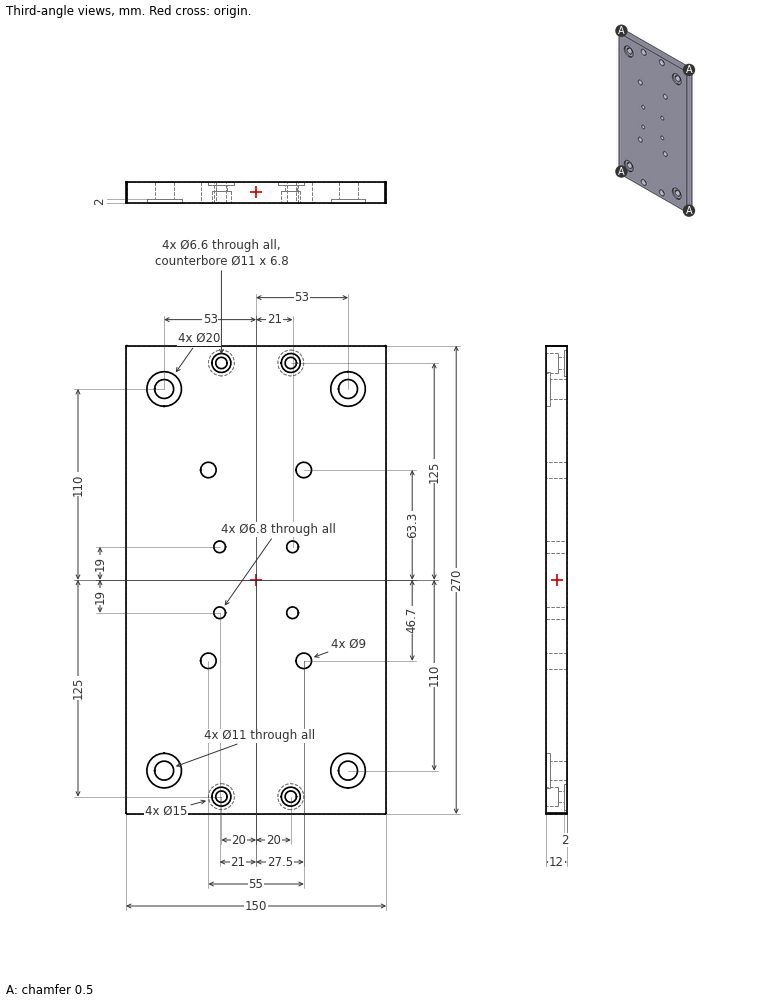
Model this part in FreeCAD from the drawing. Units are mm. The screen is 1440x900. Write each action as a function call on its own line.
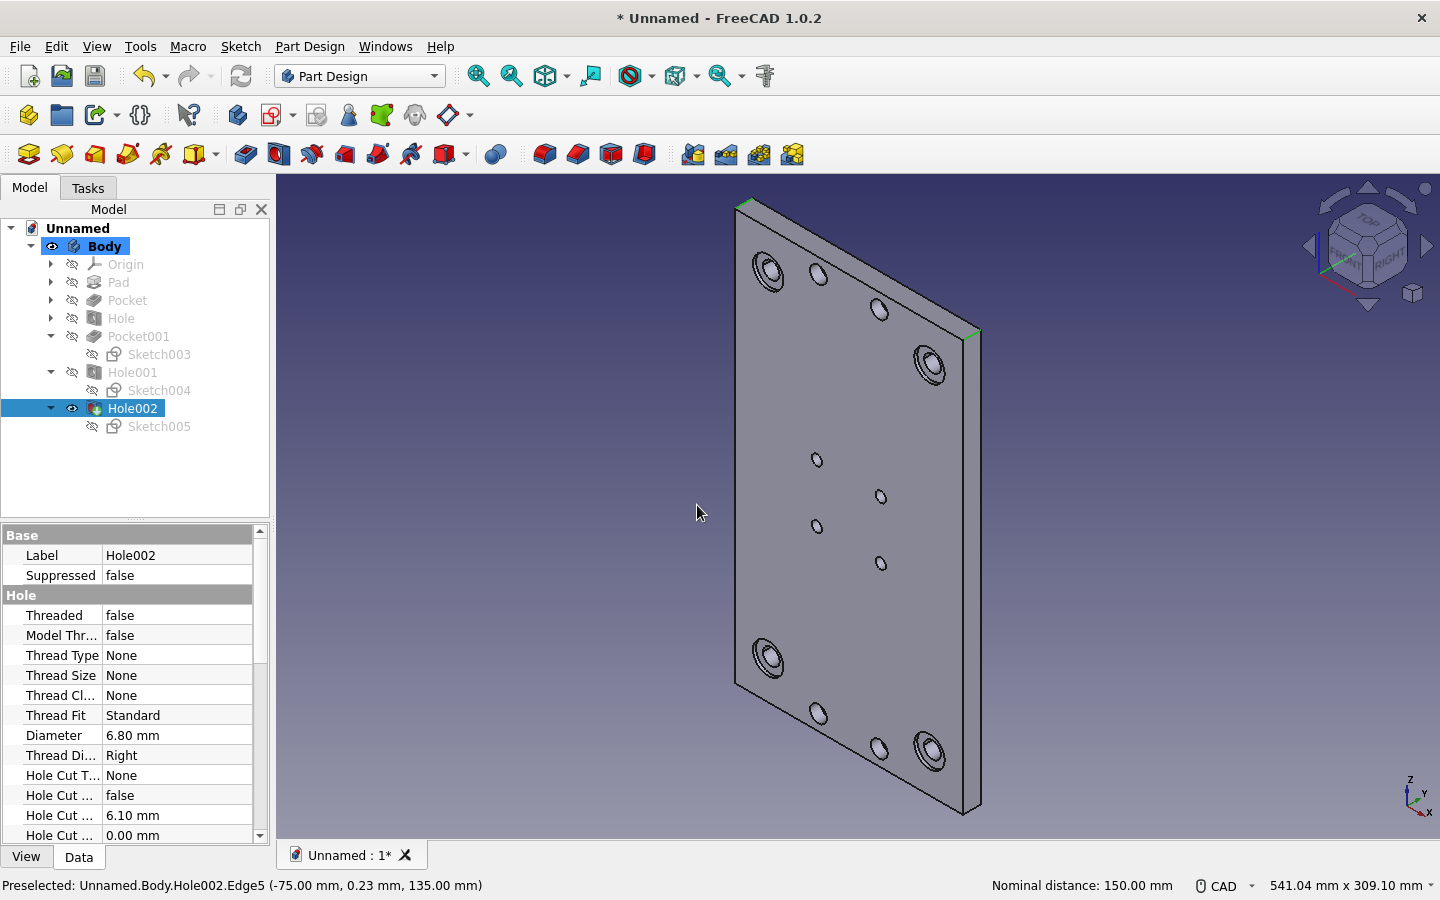
key(1)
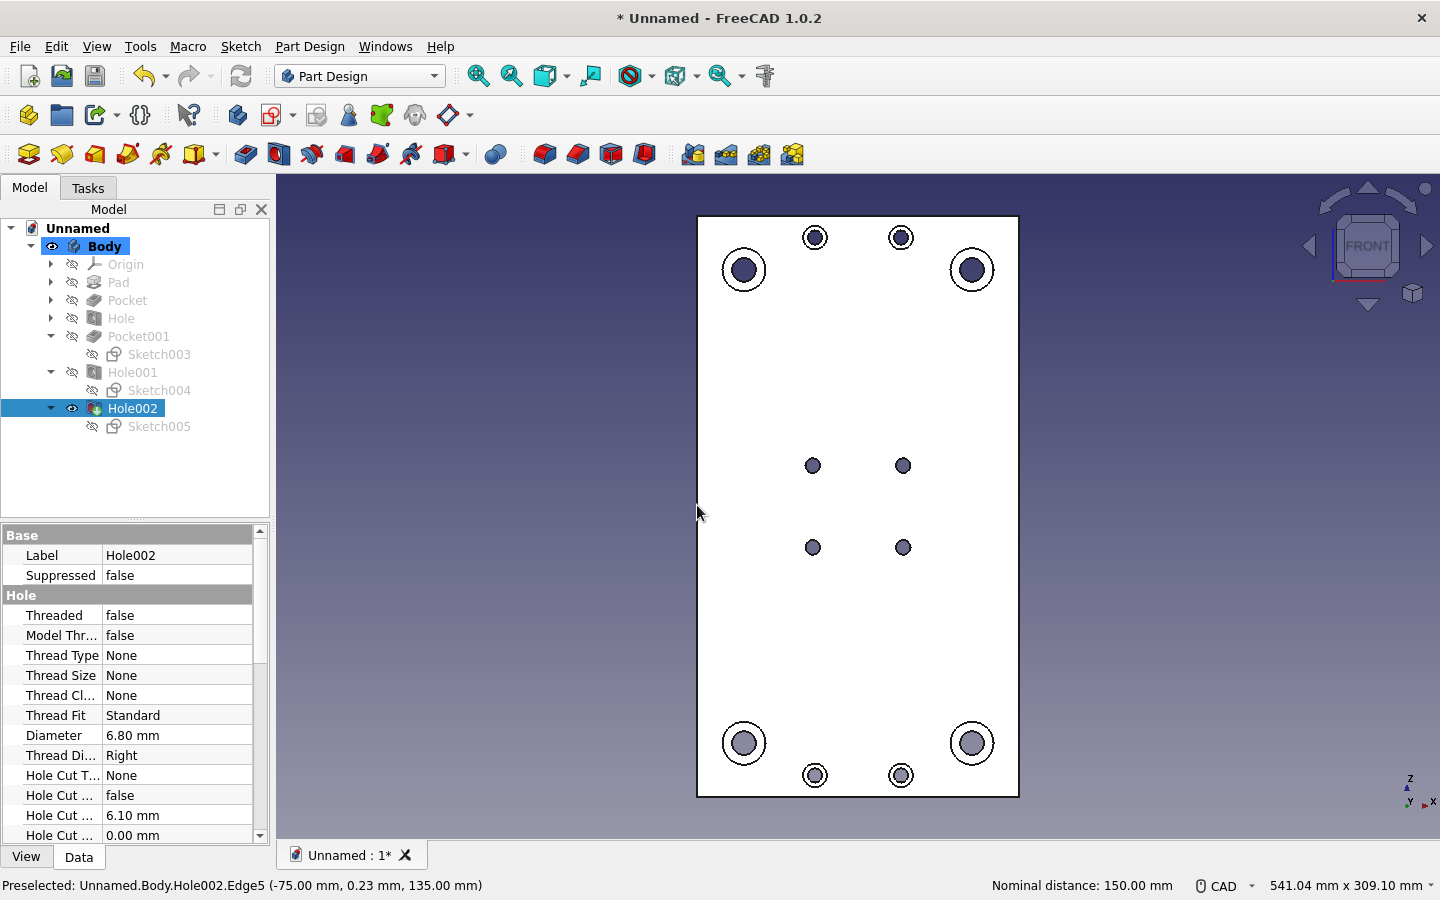
key(3)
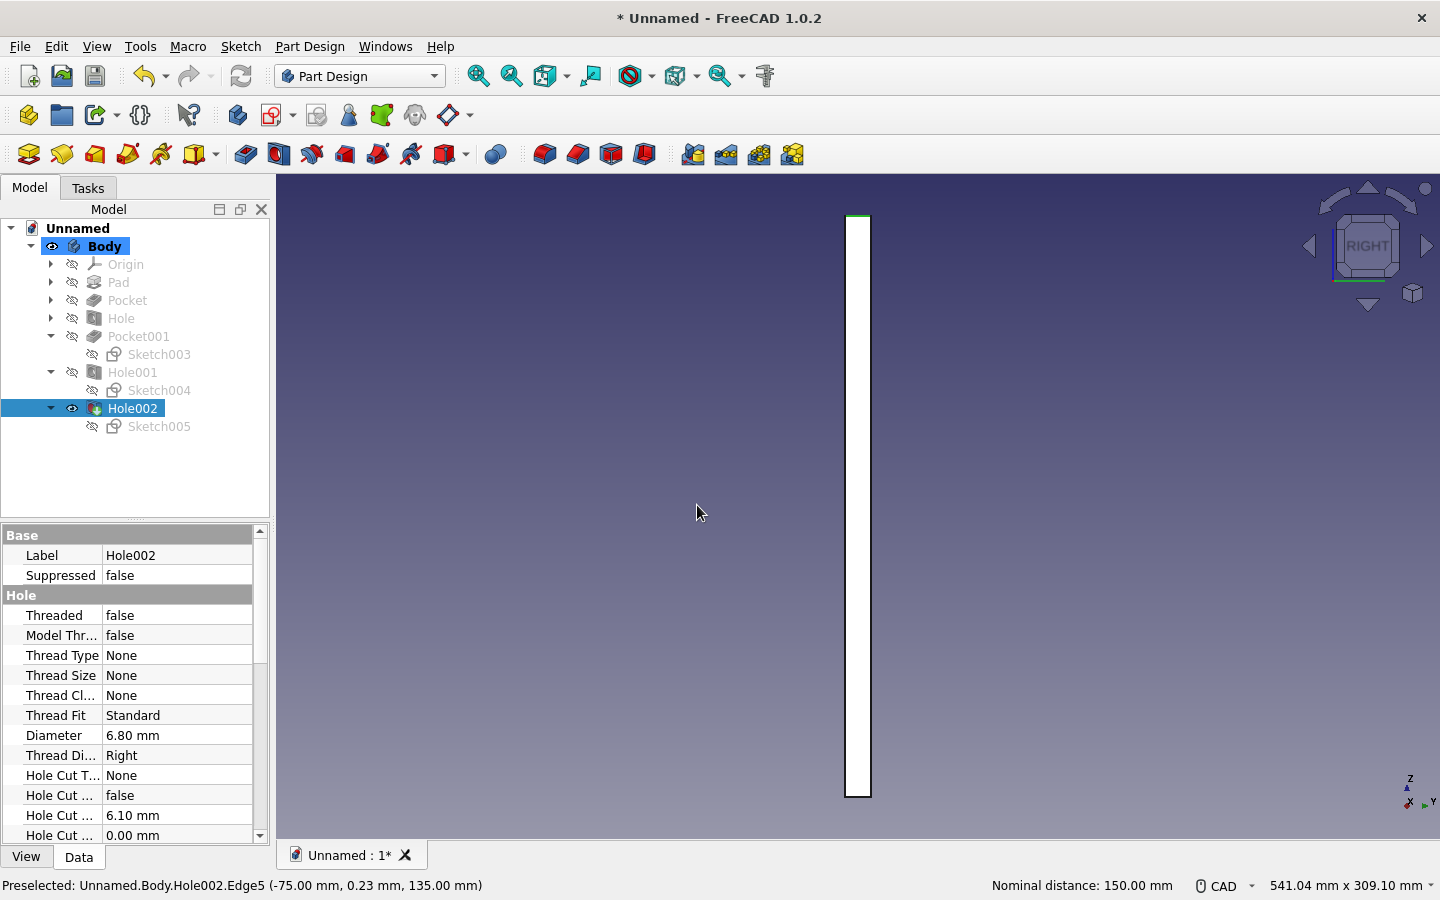
click(858, 796, ctrl)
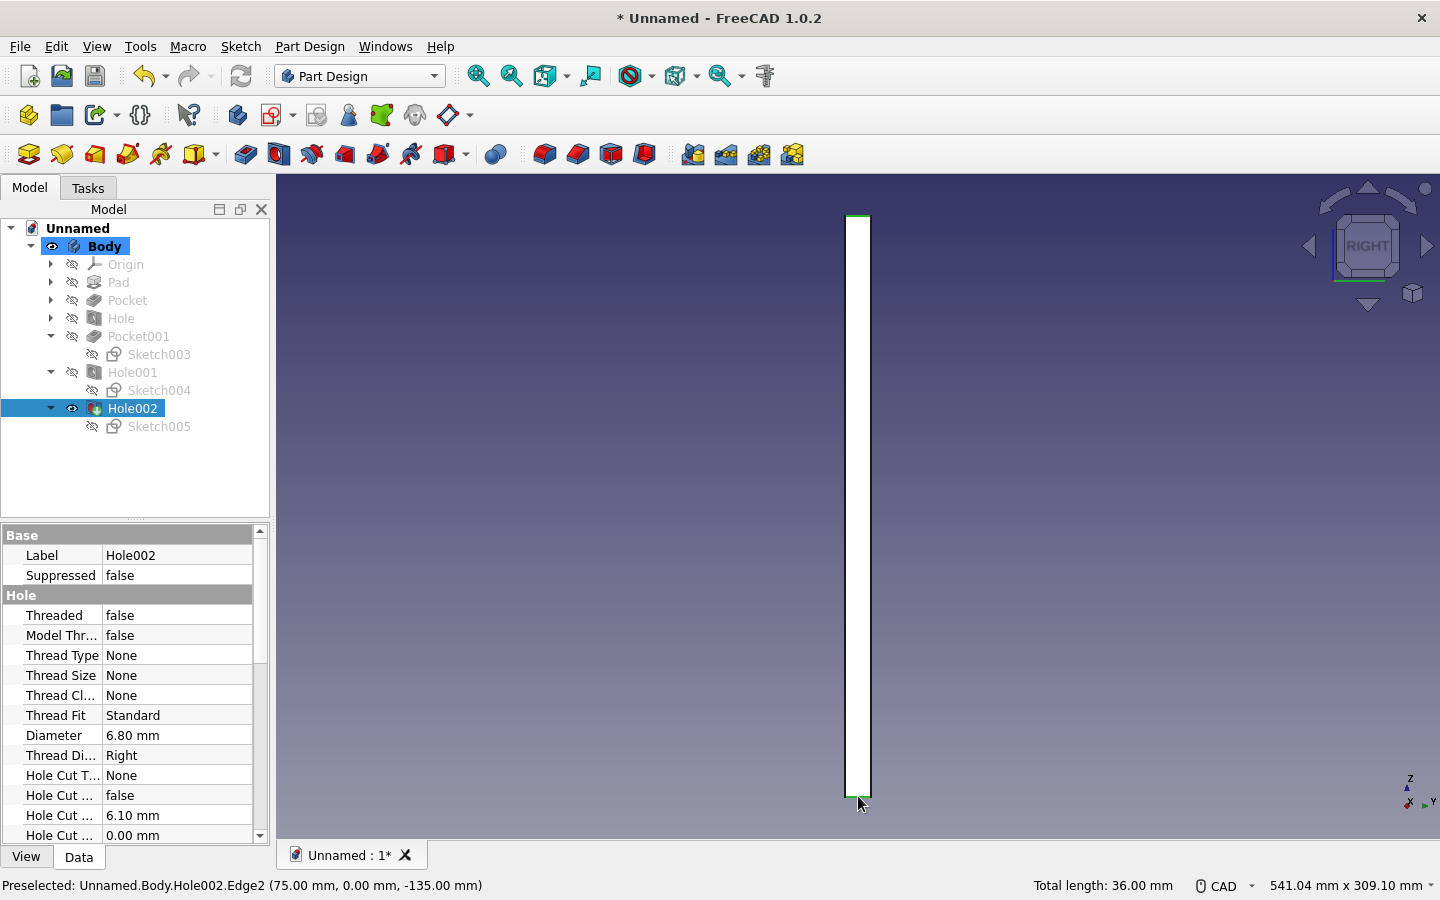
key(5)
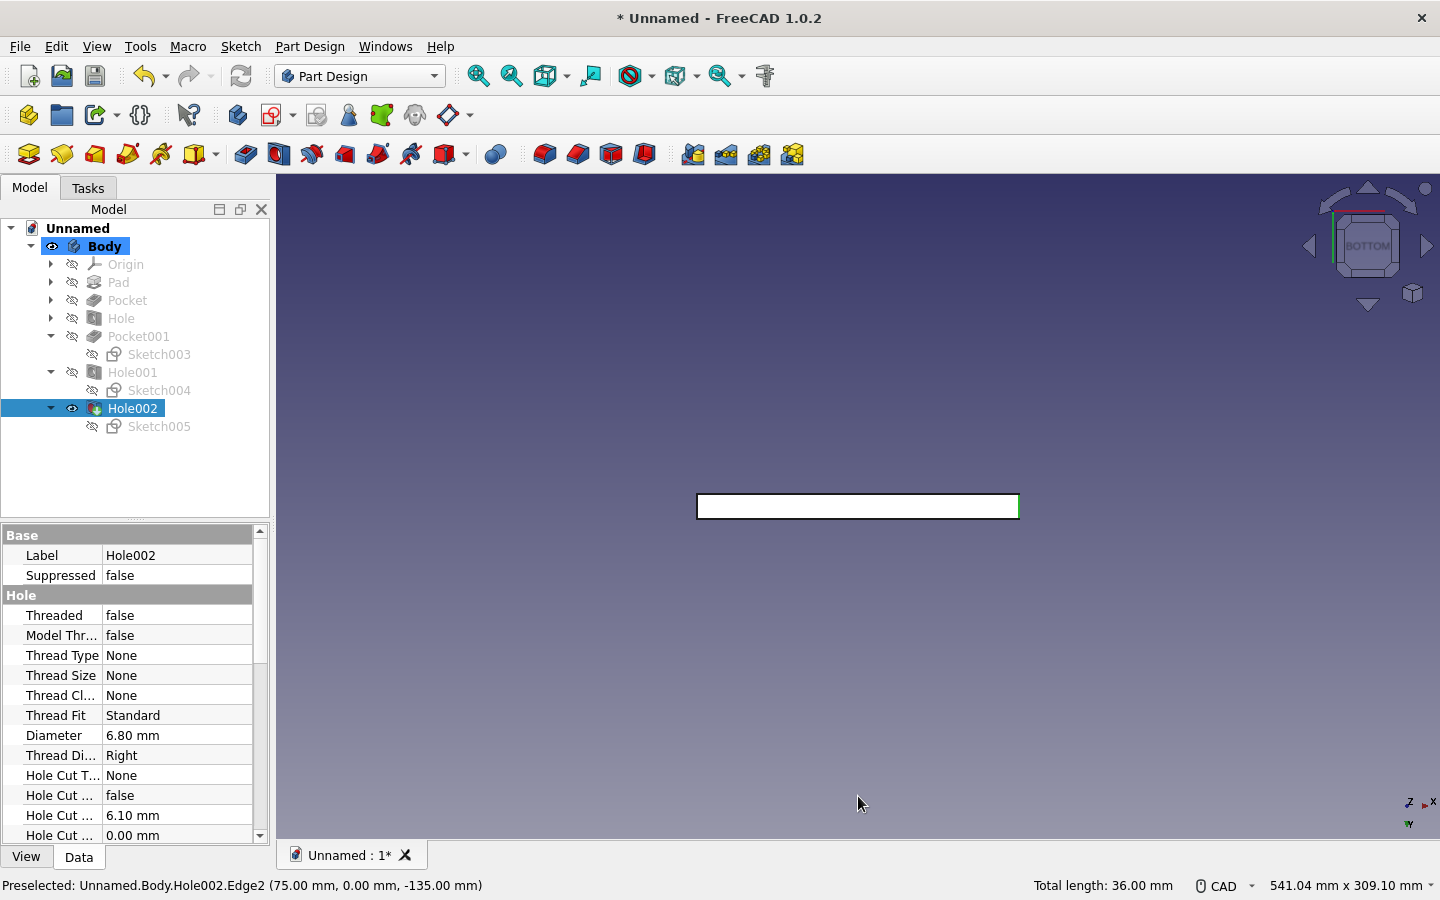
key(v)
key(f)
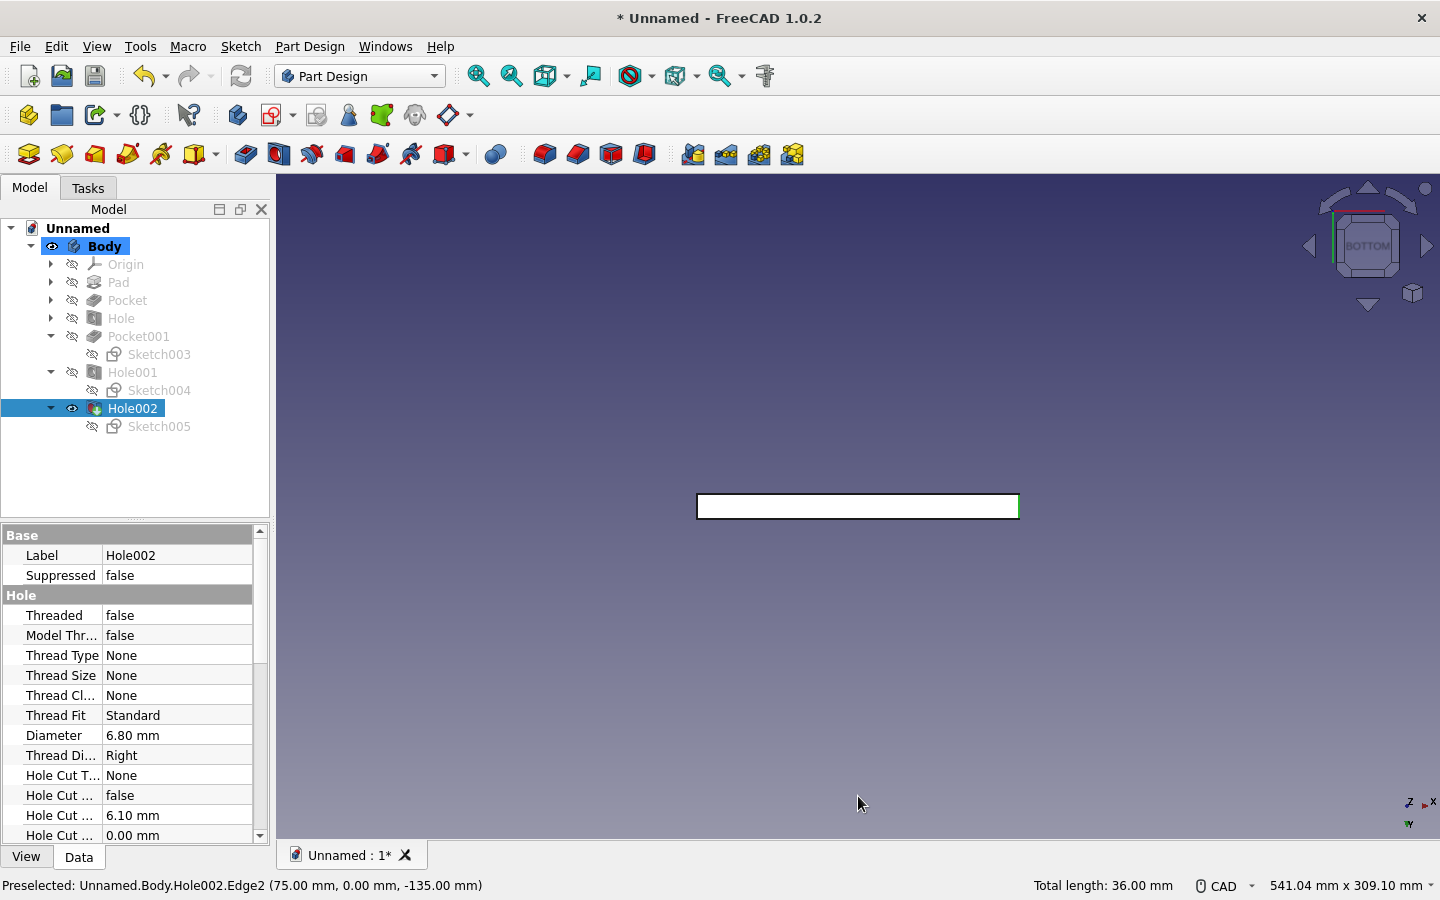
click(697, 505, ctrl)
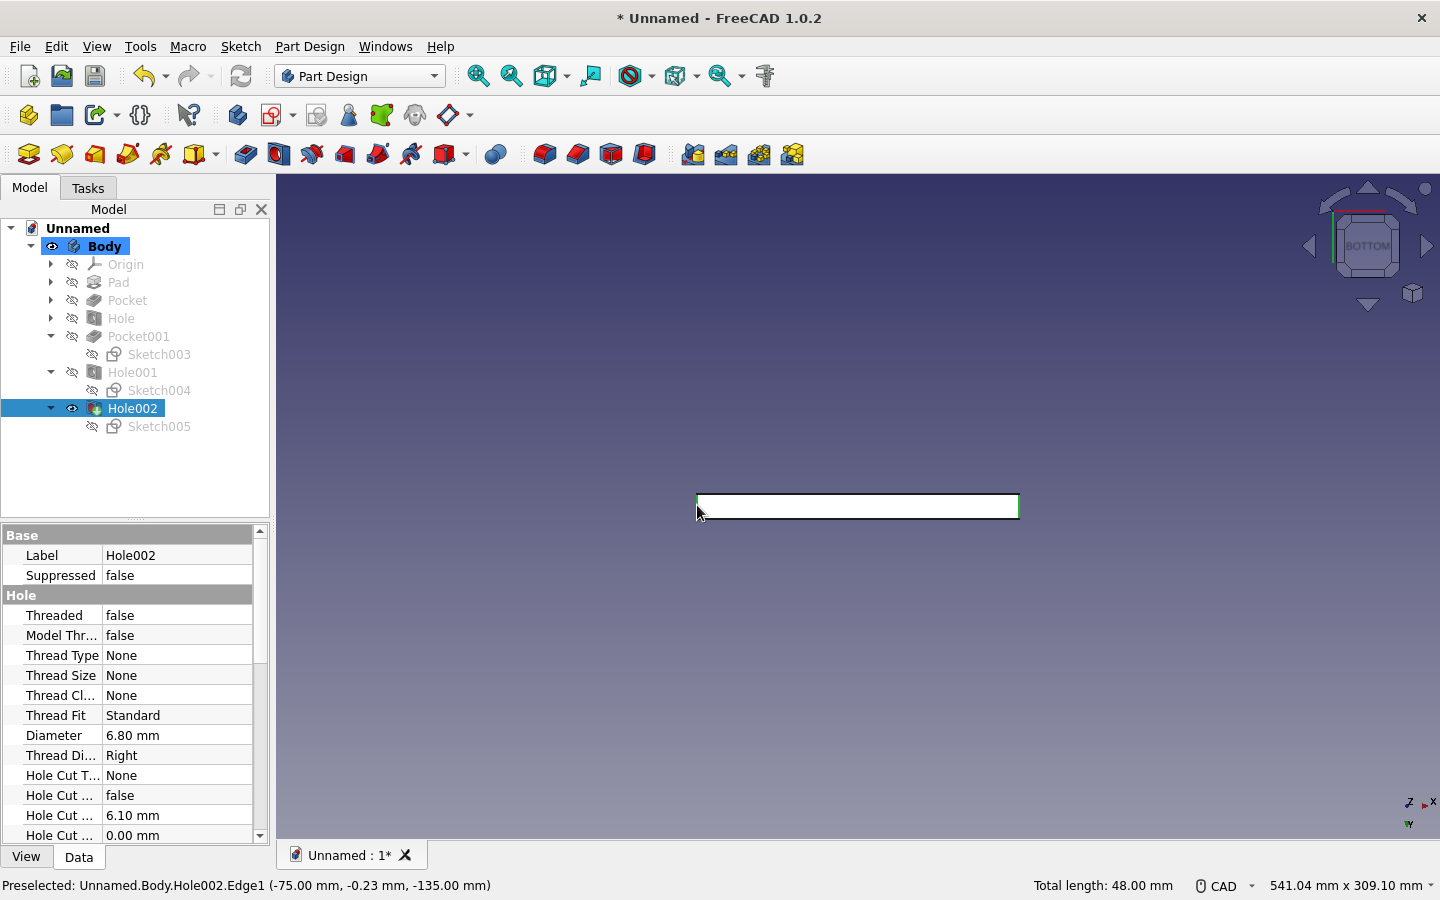
click(578, 154)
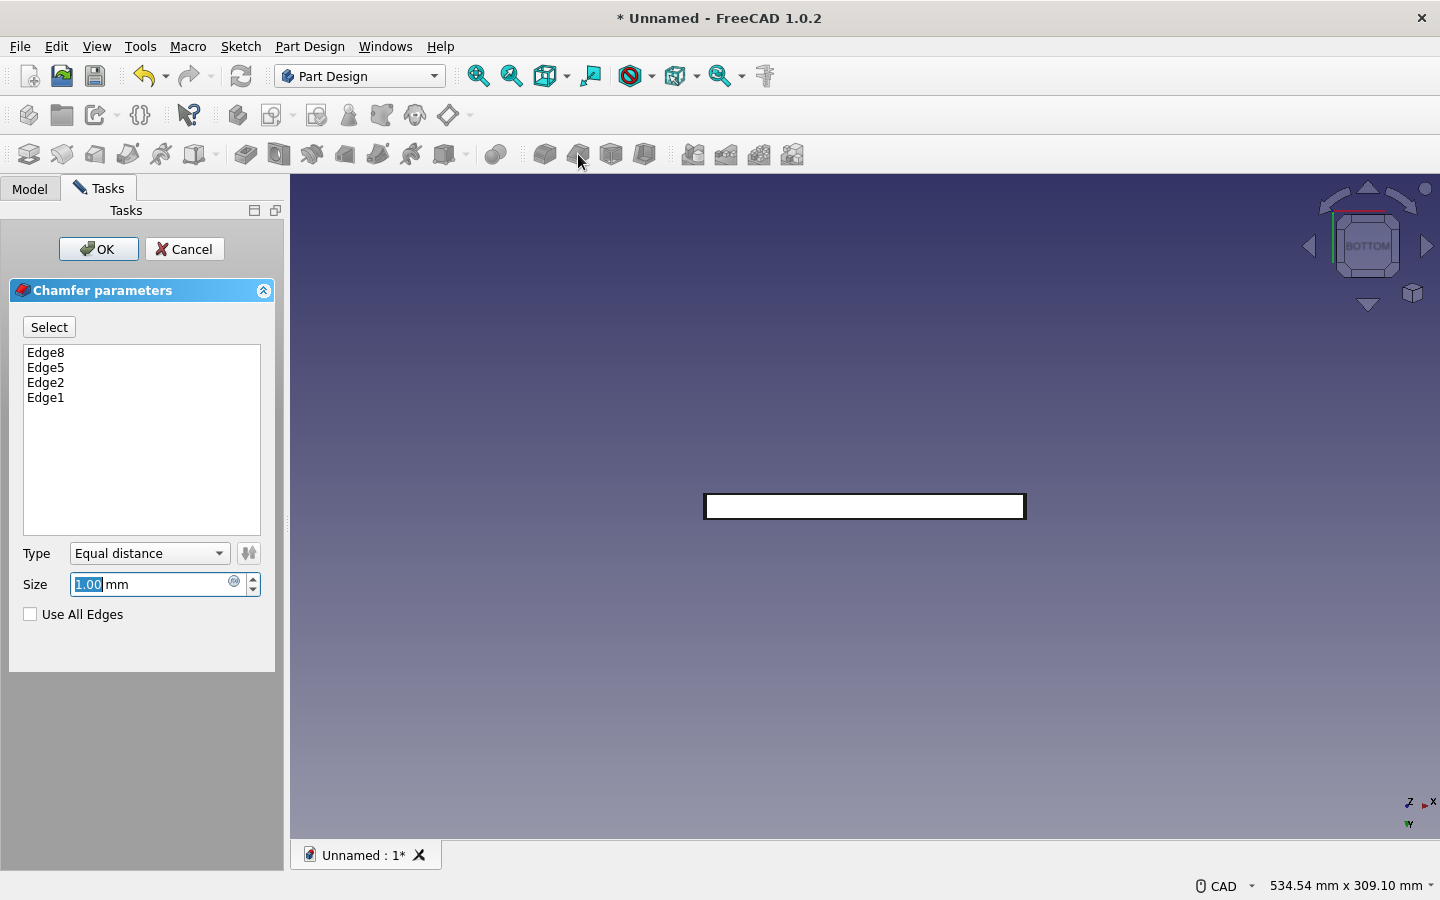
text(0.5)
key(Tab)